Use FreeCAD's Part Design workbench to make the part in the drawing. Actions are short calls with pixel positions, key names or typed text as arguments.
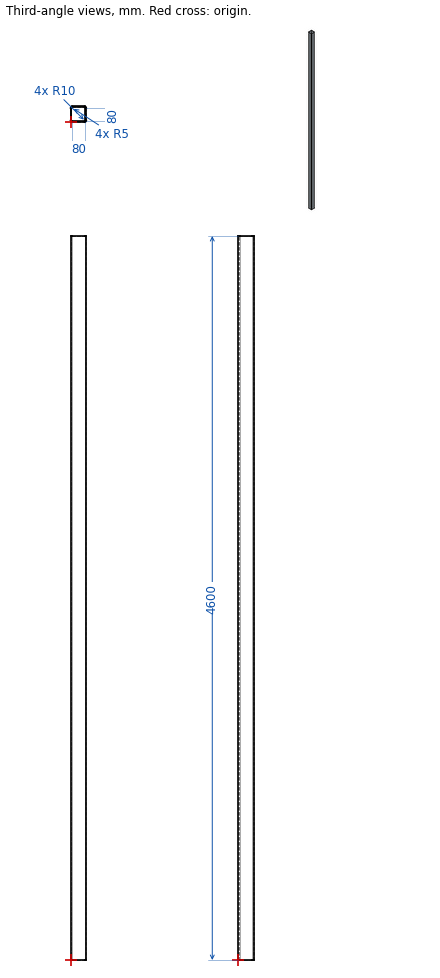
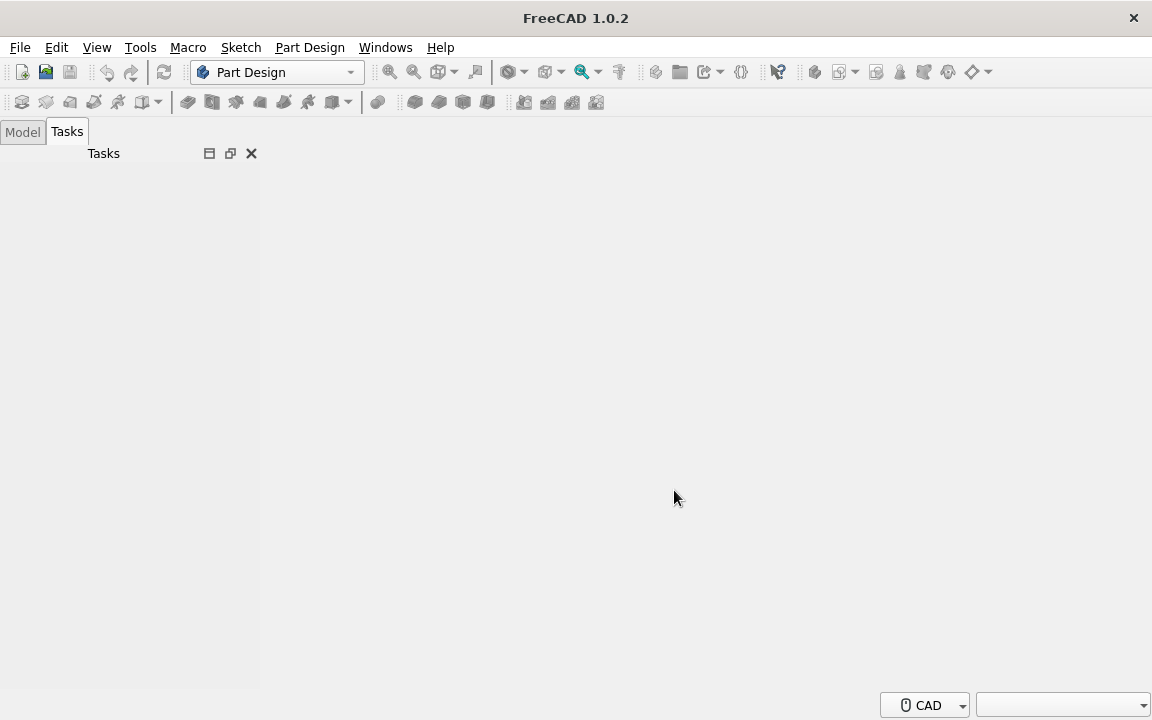
click(22, 72)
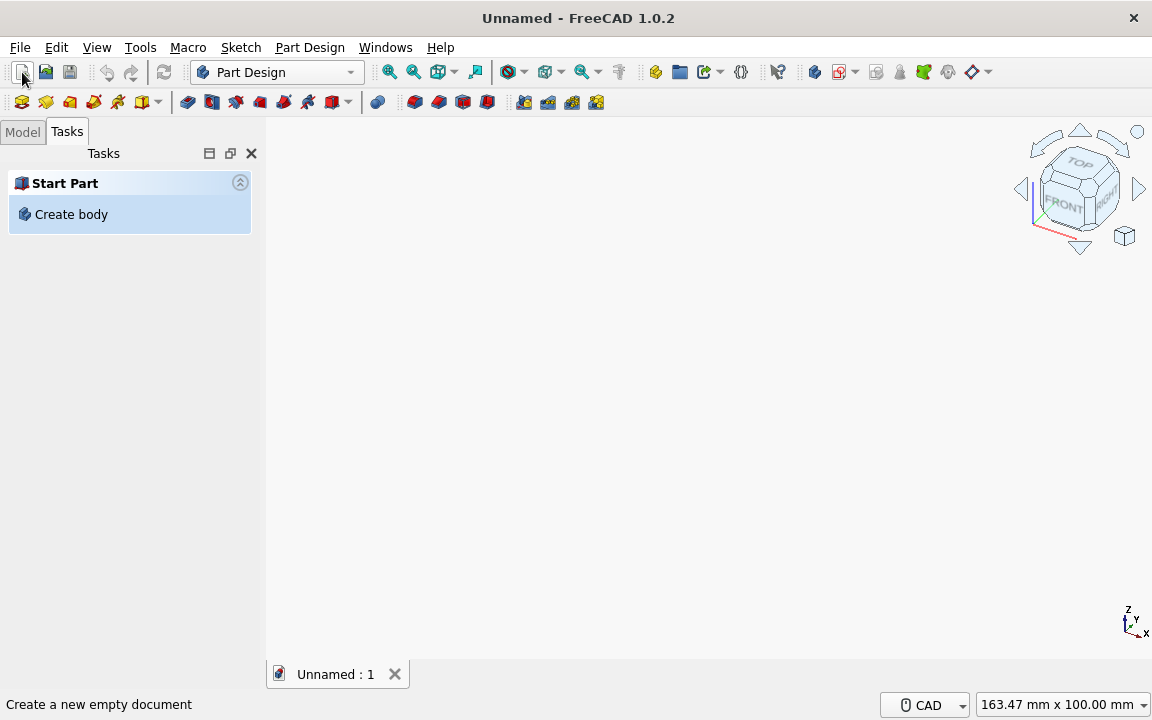
click(840, 72)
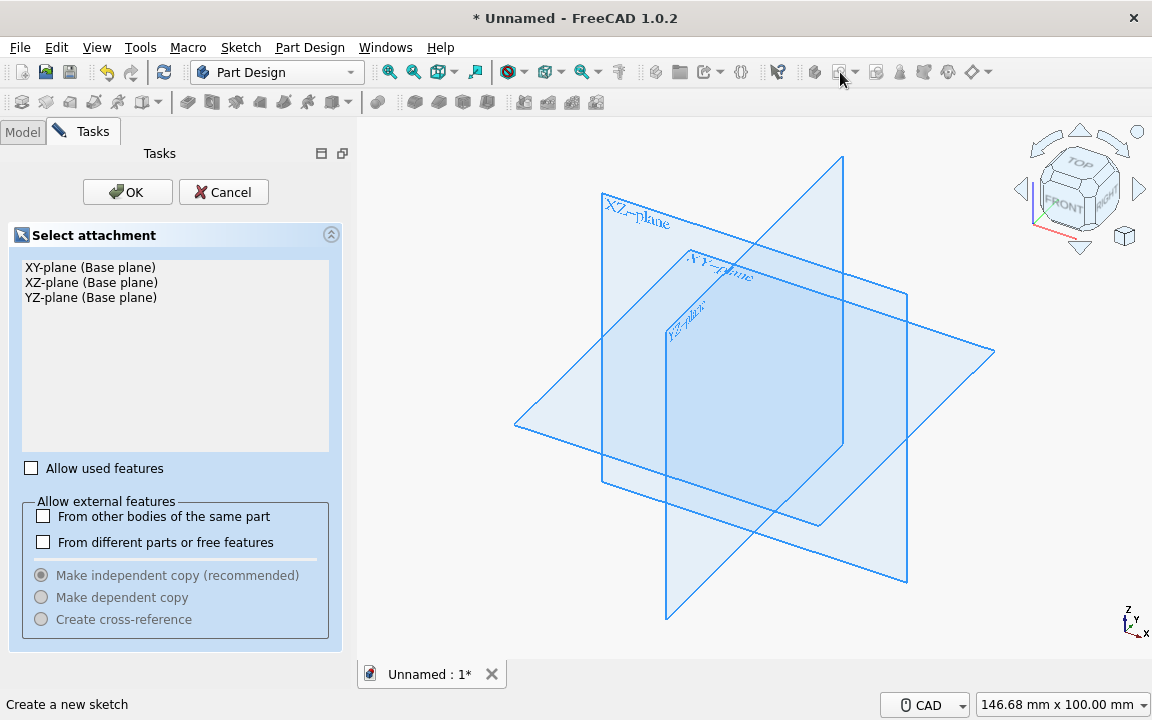
click(82, 268)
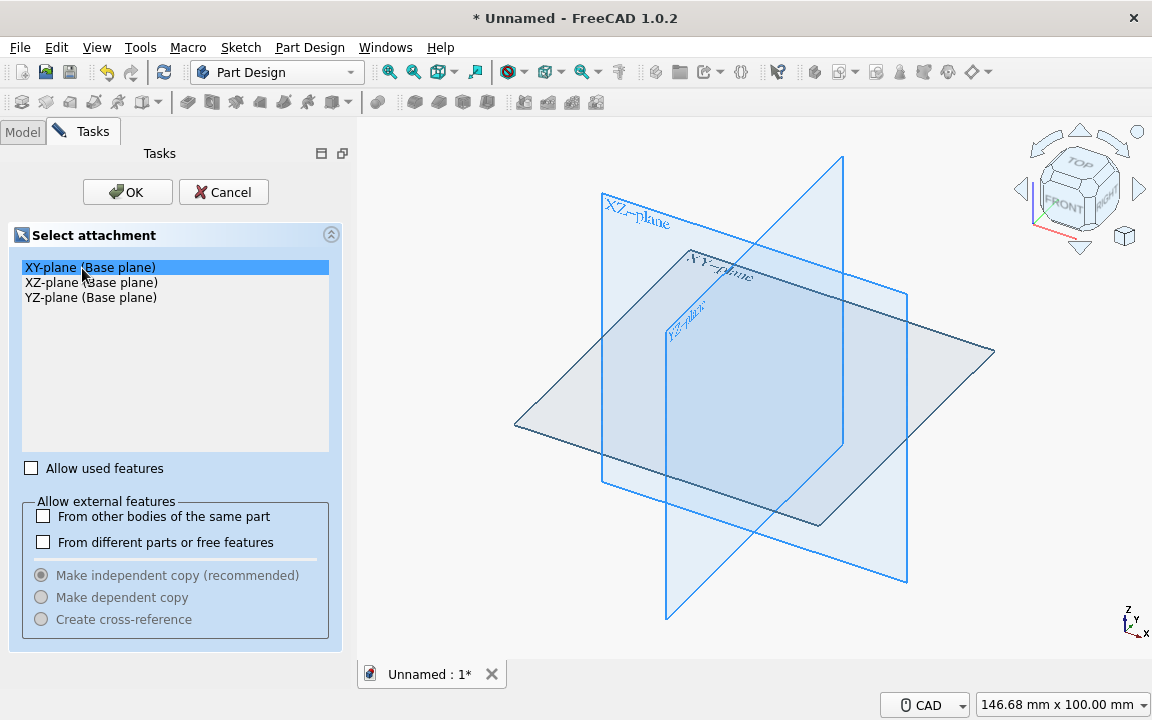
click(128, 192)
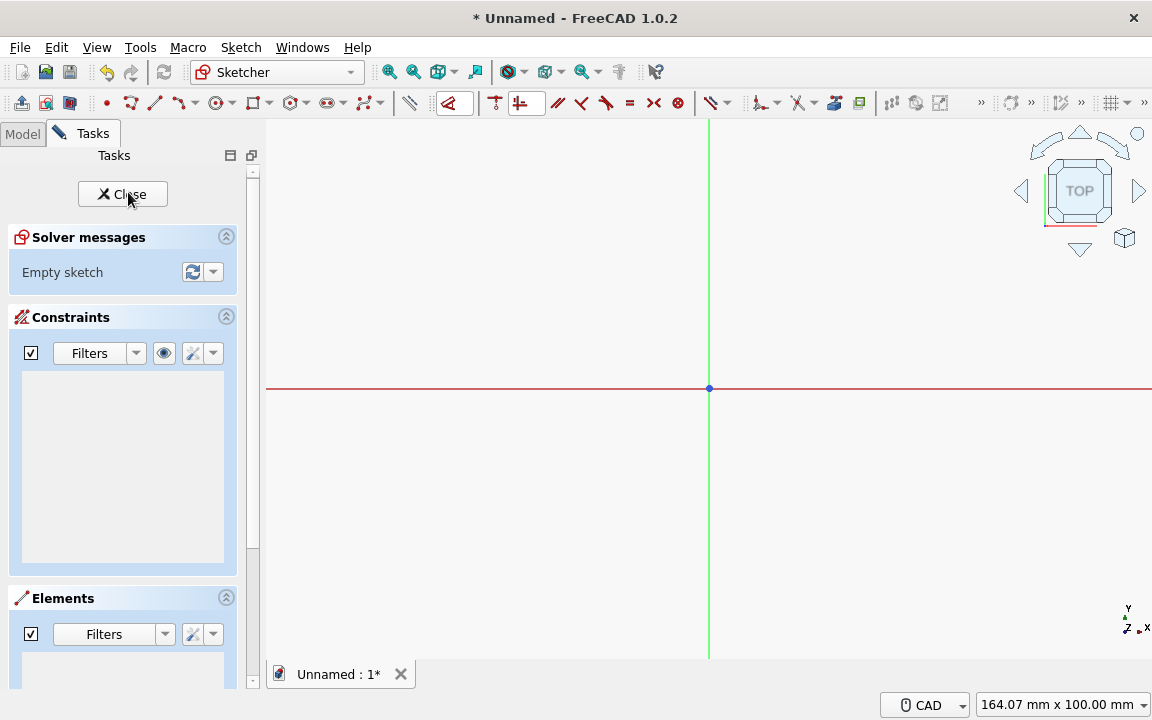
scroll(294, 631, down, 3)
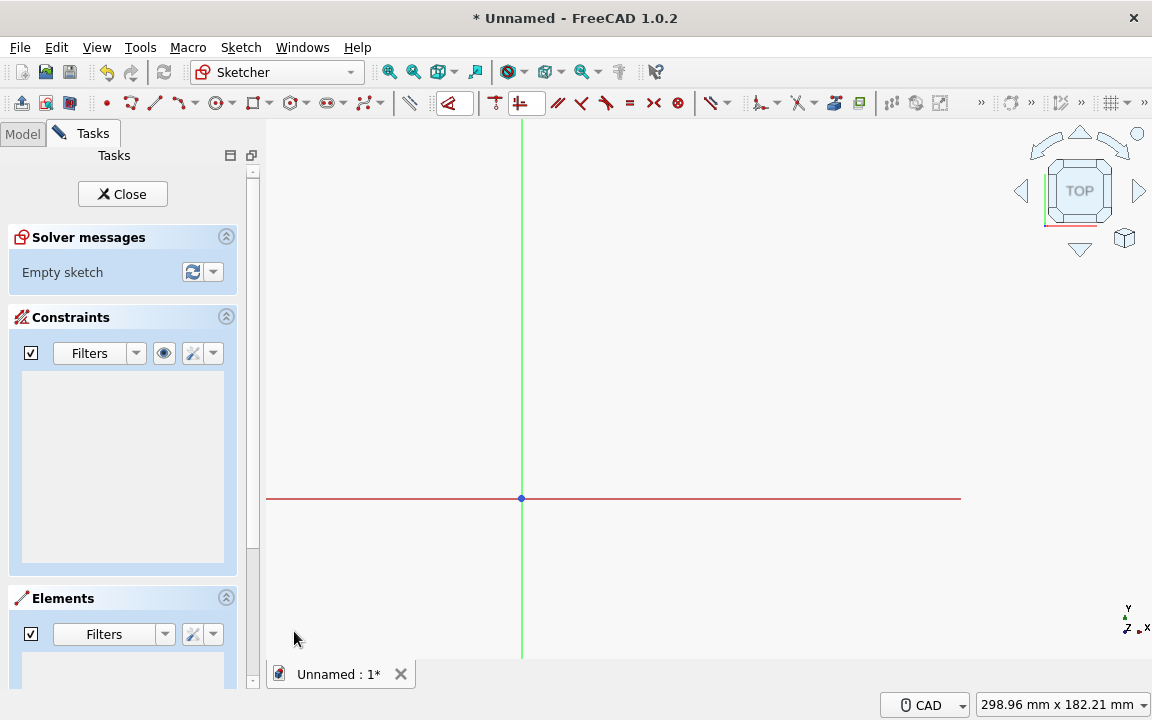
click(156, 104)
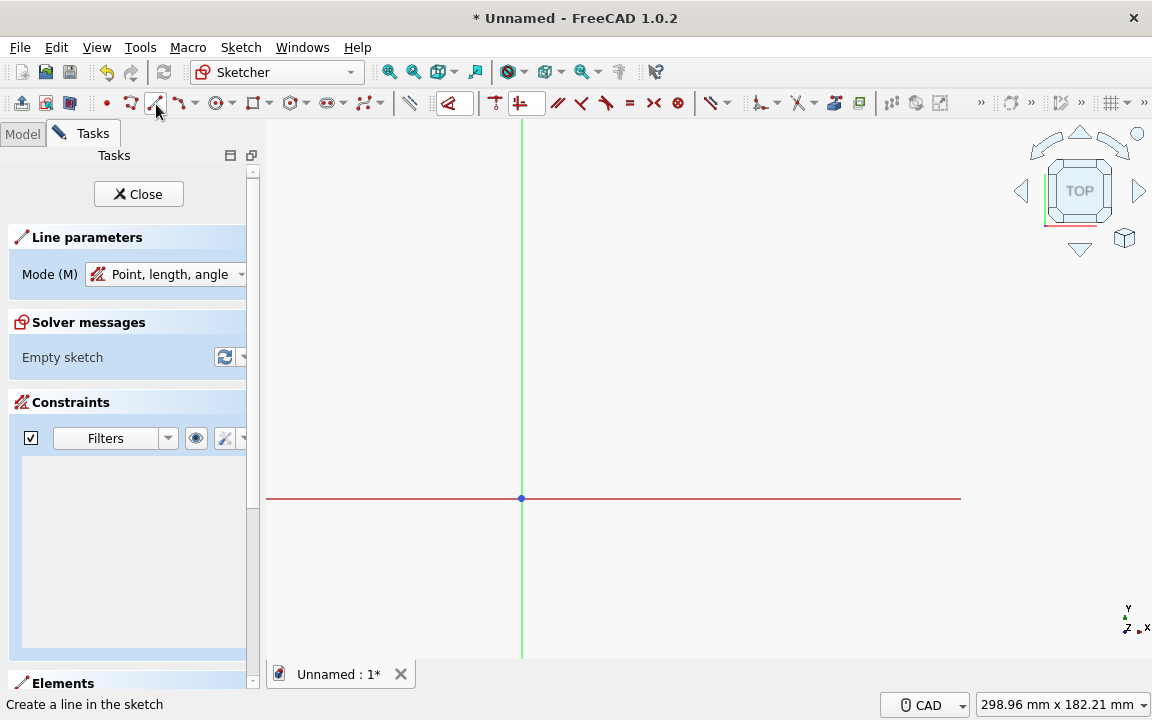
click(551, 499)
click(788, 490)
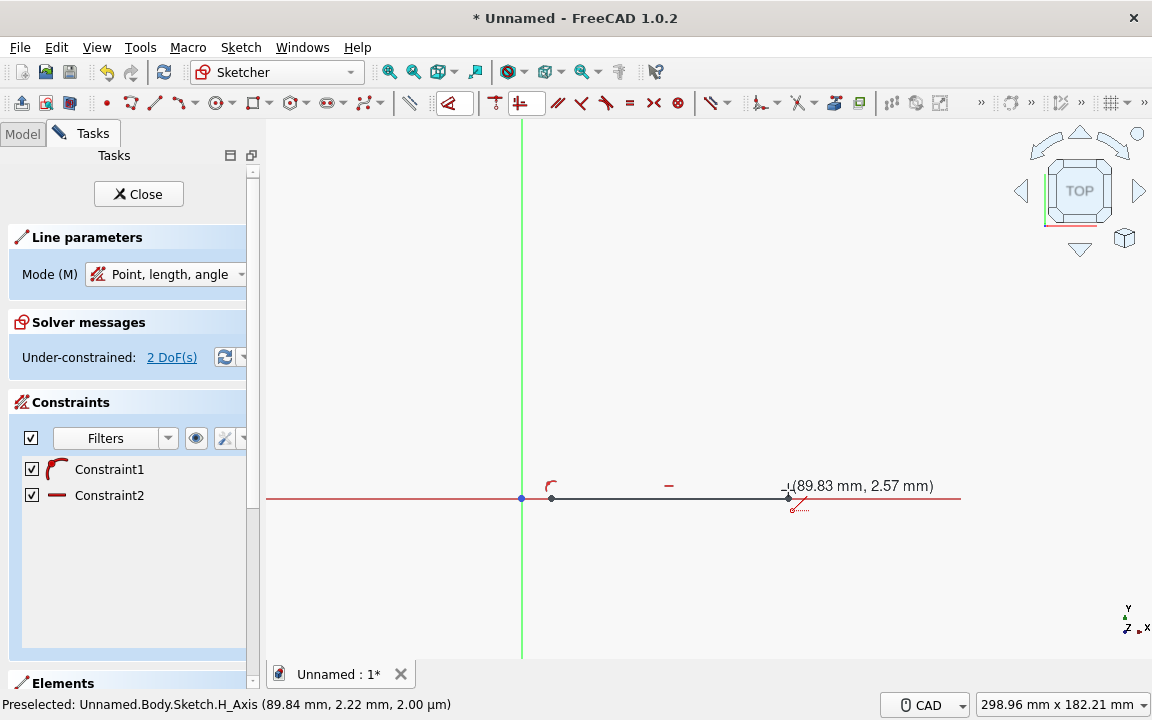
click(818, 469)
click(818, 232)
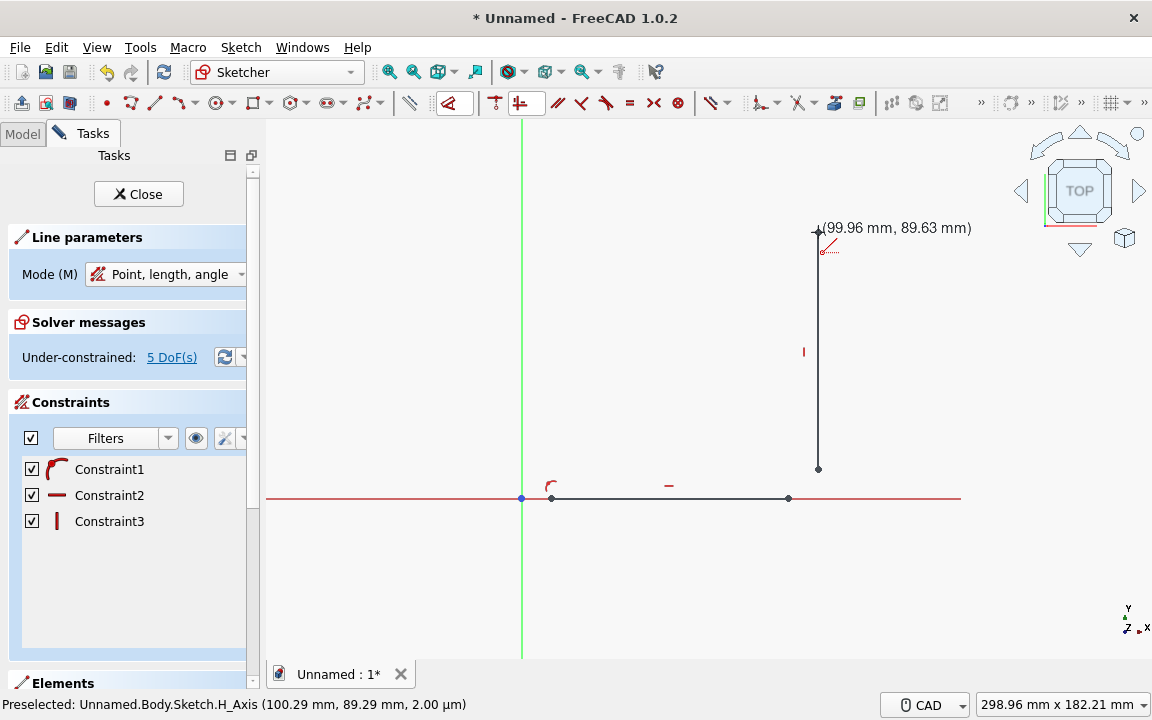
click(788, 202)
click(551, 202)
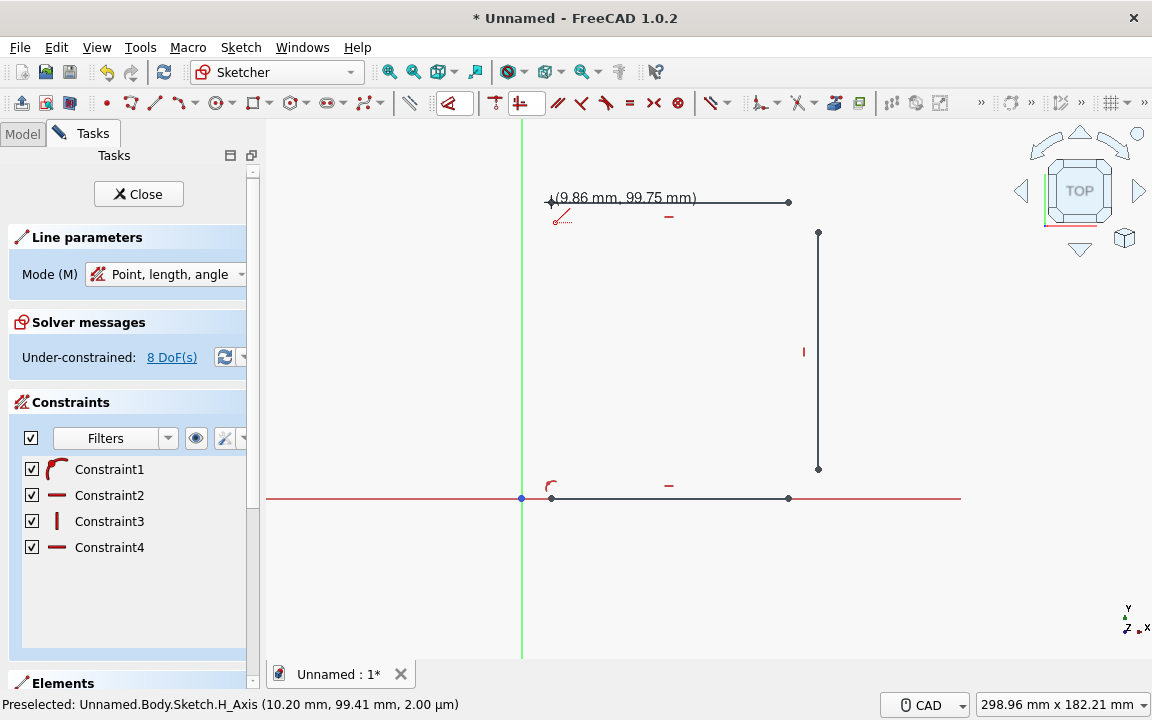
click(522, 232)
click(531, 469)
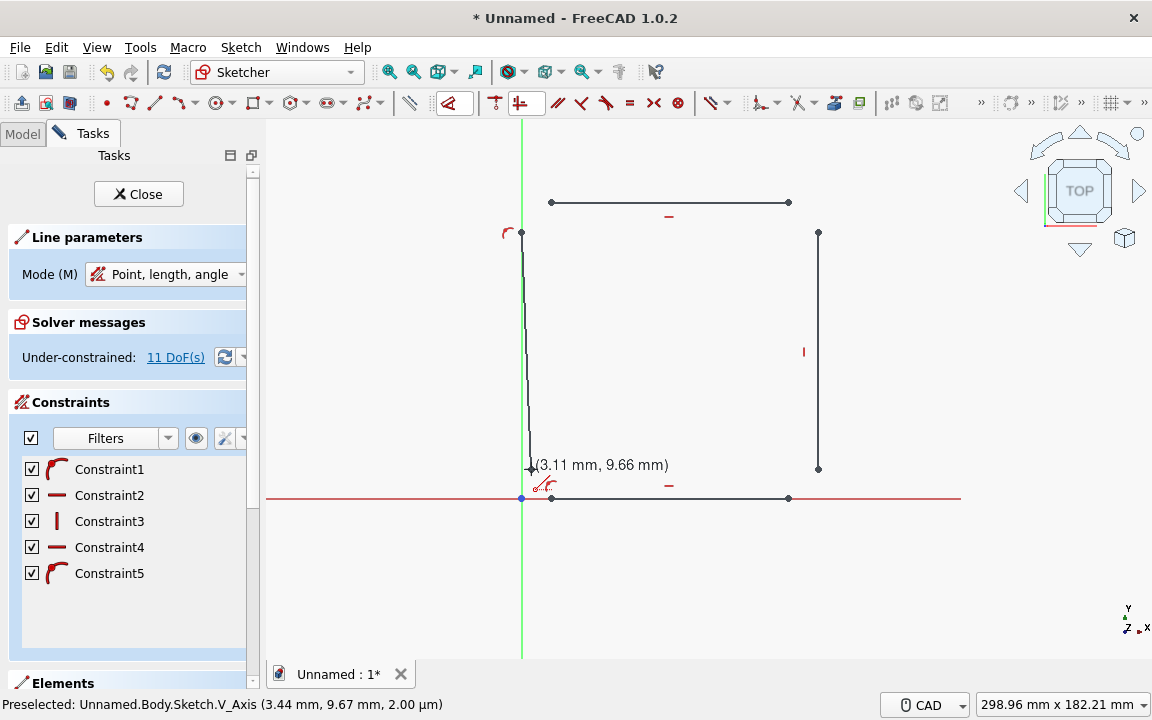
click(180, 104)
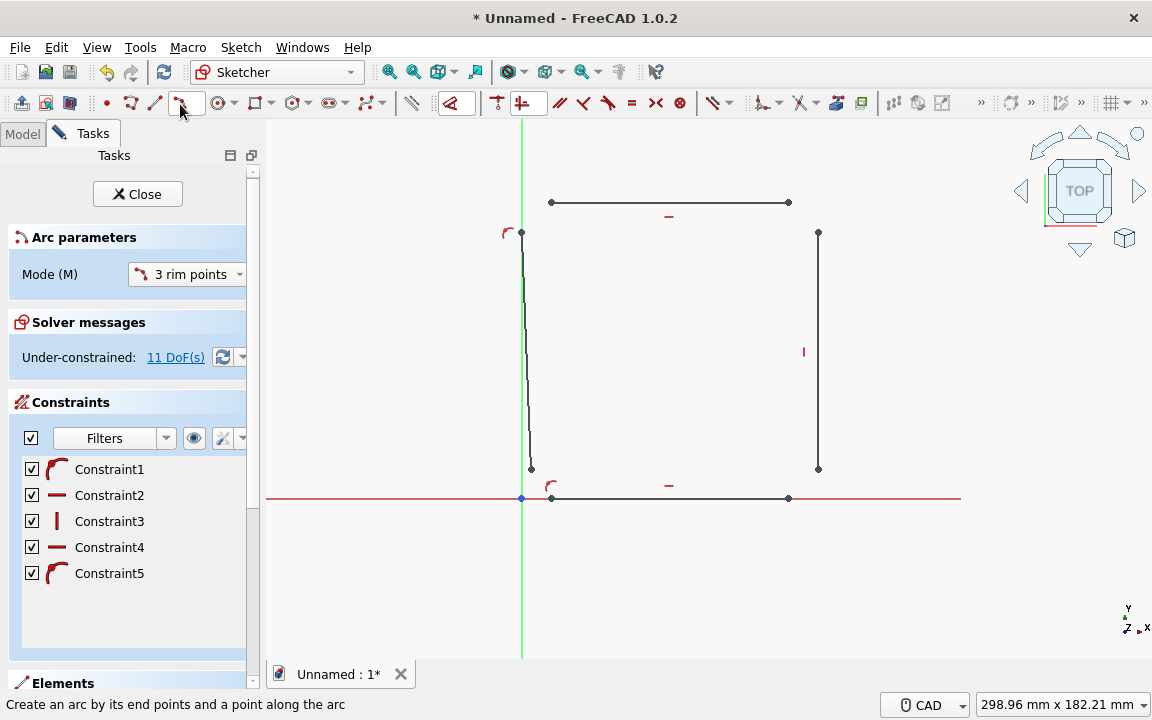
click(788, 499)
click(818, 470)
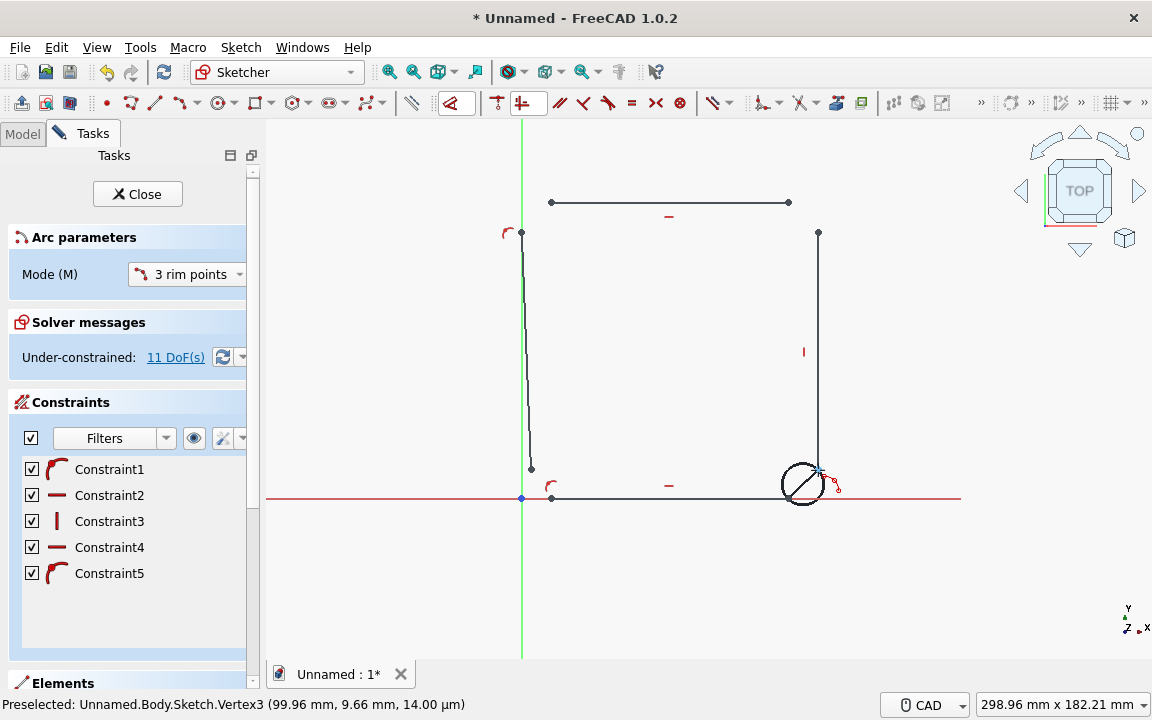
scroll(809, 490, up, 4)